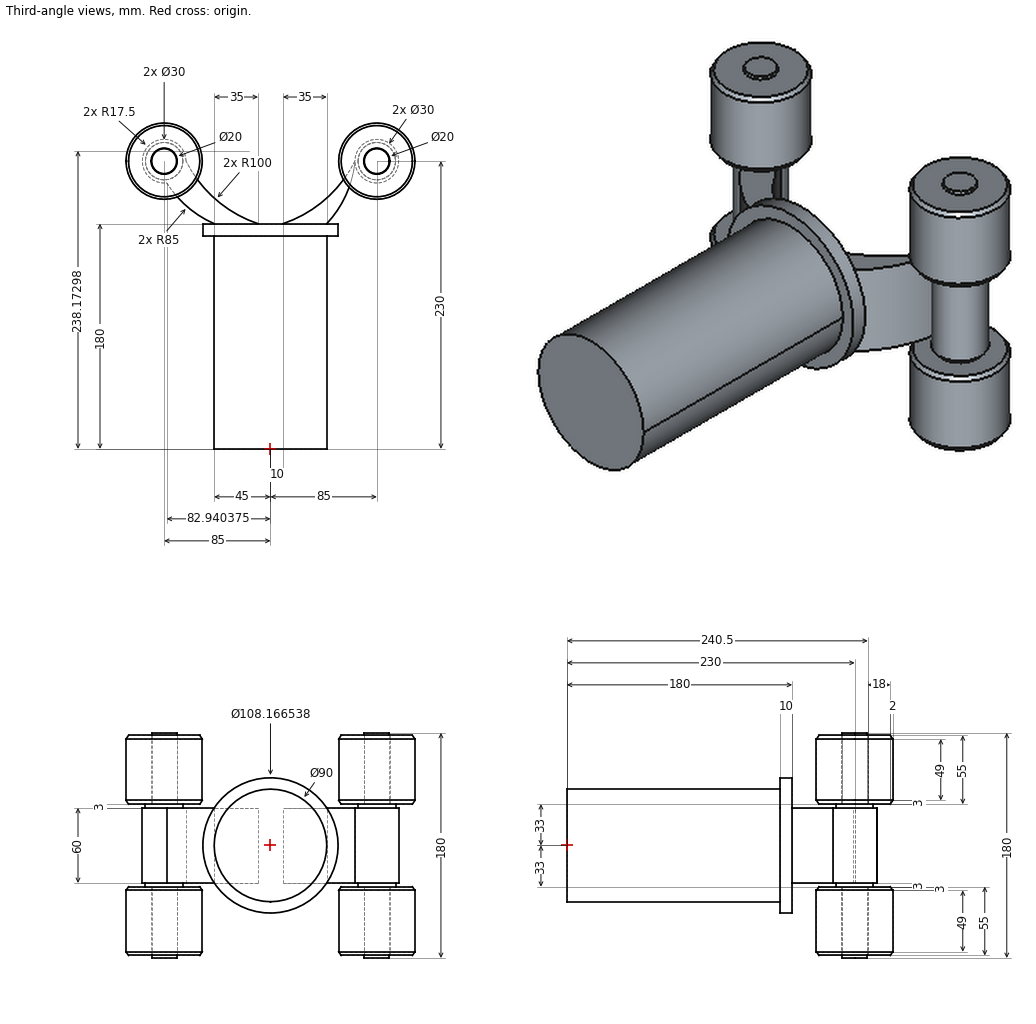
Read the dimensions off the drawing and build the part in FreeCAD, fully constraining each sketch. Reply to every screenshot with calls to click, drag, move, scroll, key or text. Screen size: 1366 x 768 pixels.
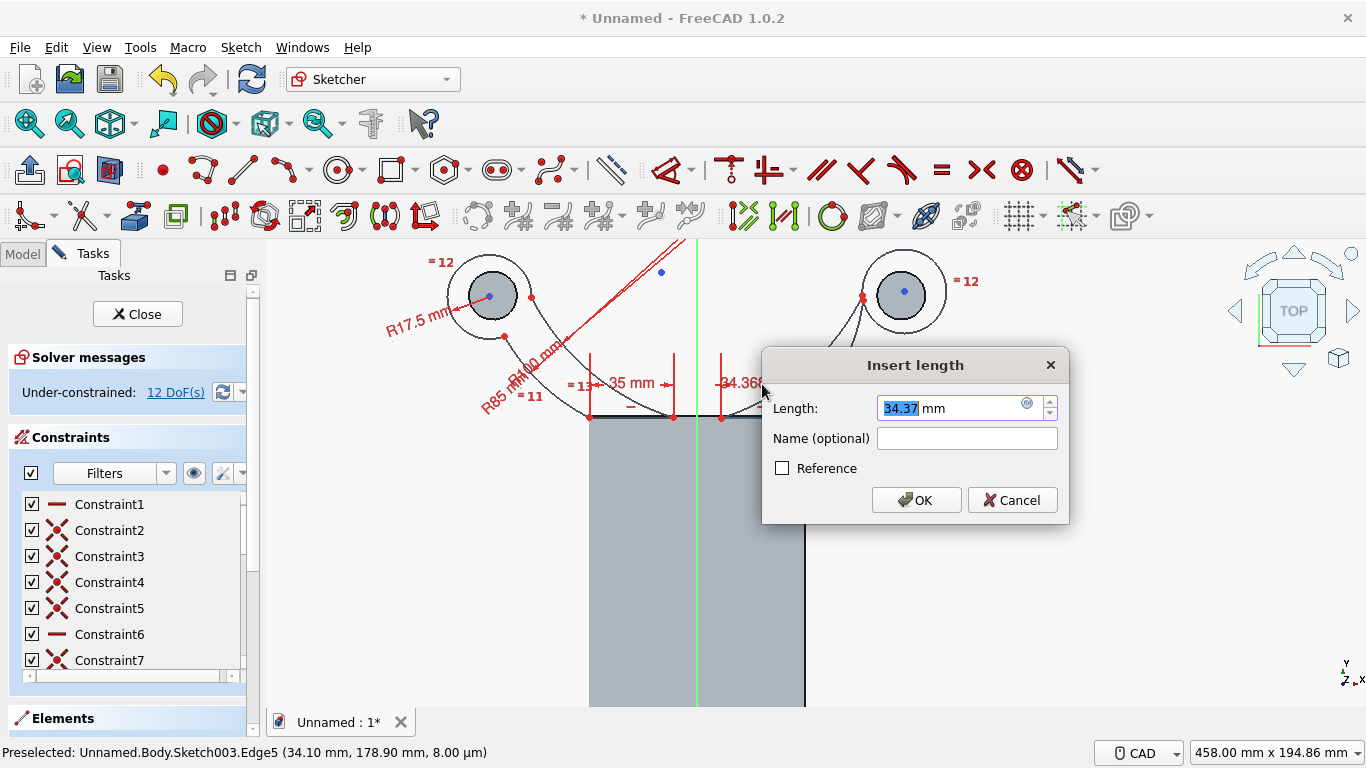
text(35)
key(Return)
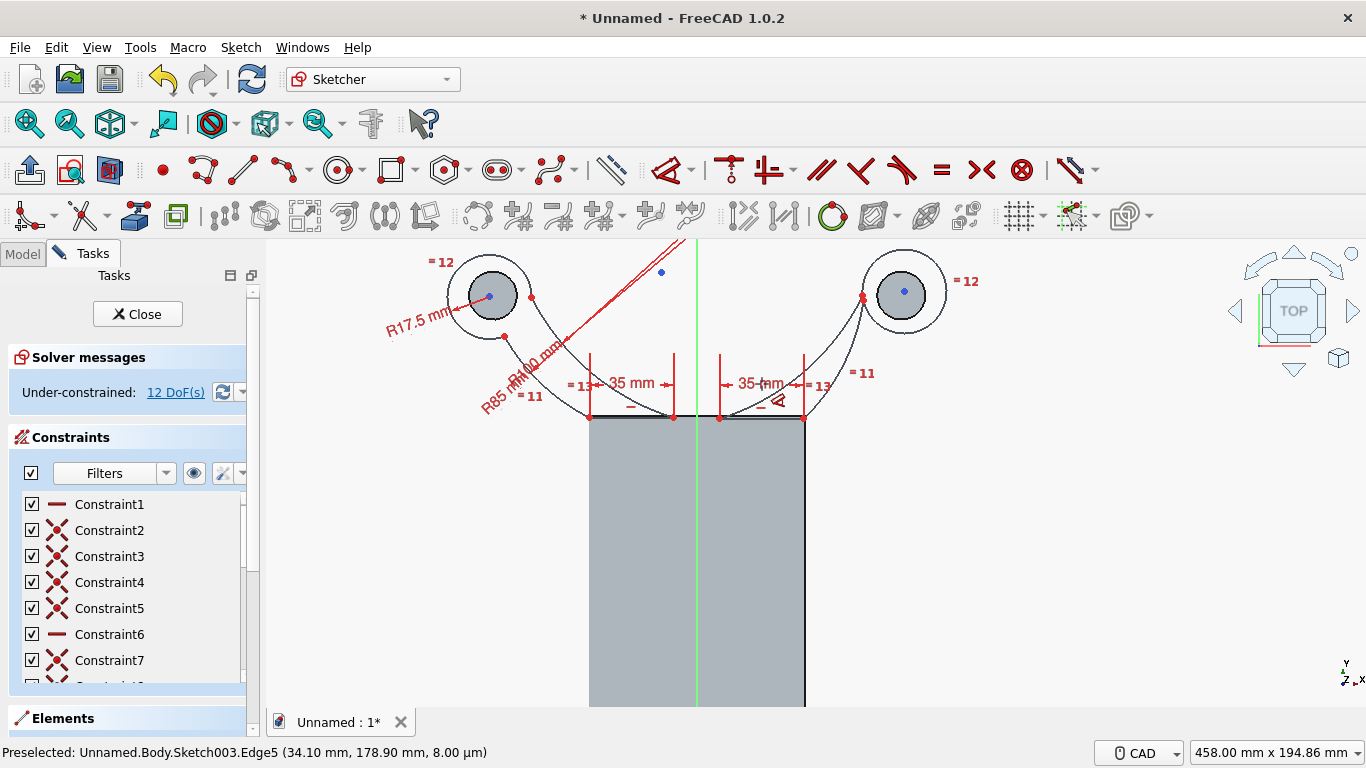
click(590, 418)
click(643, 360)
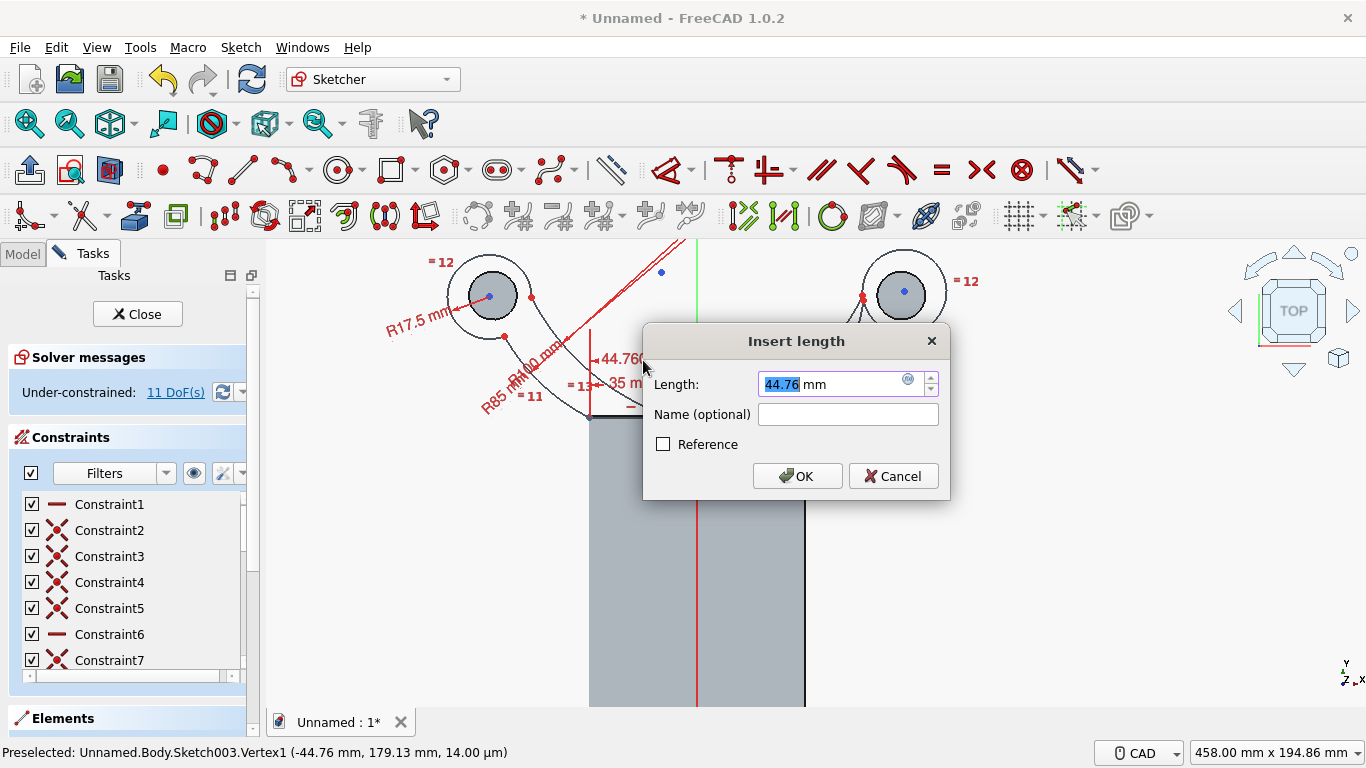
text(45)
key(Return)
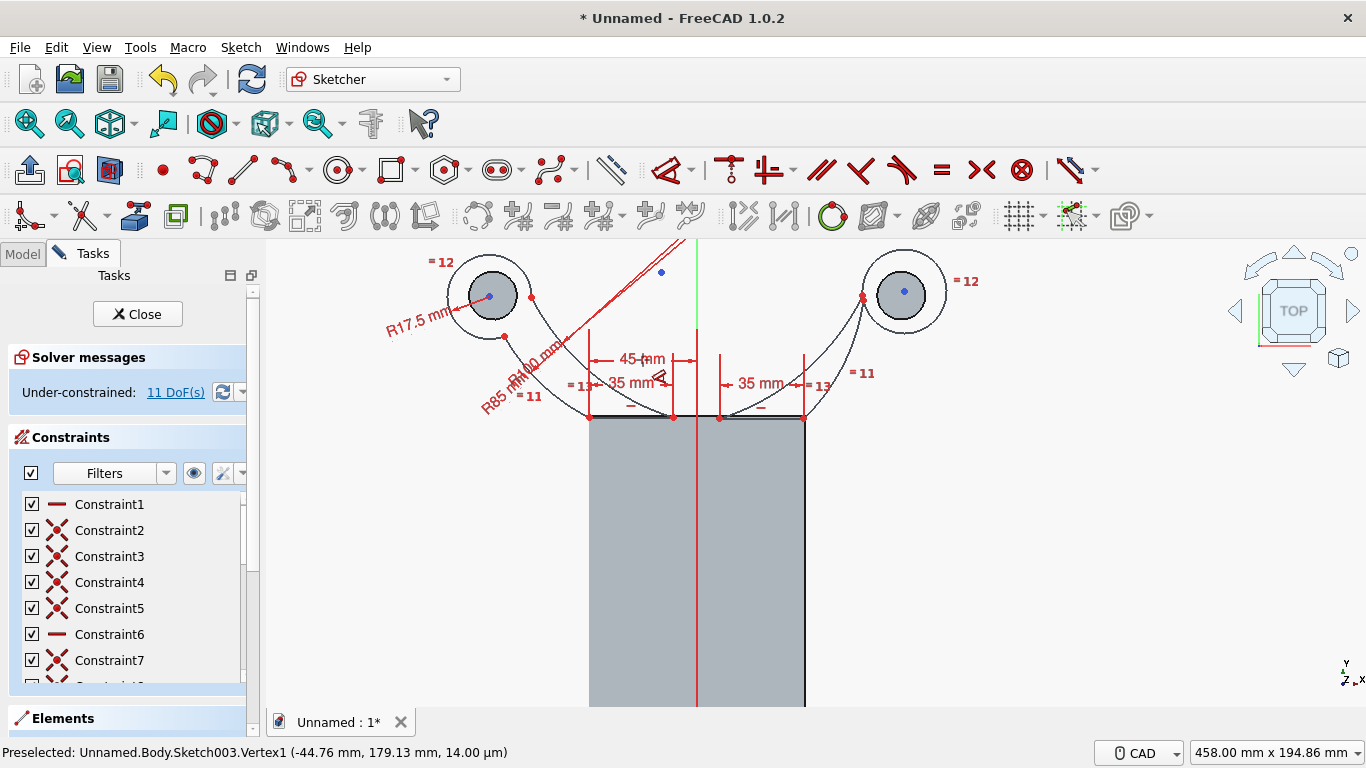
scroll(720, 419, up, 3)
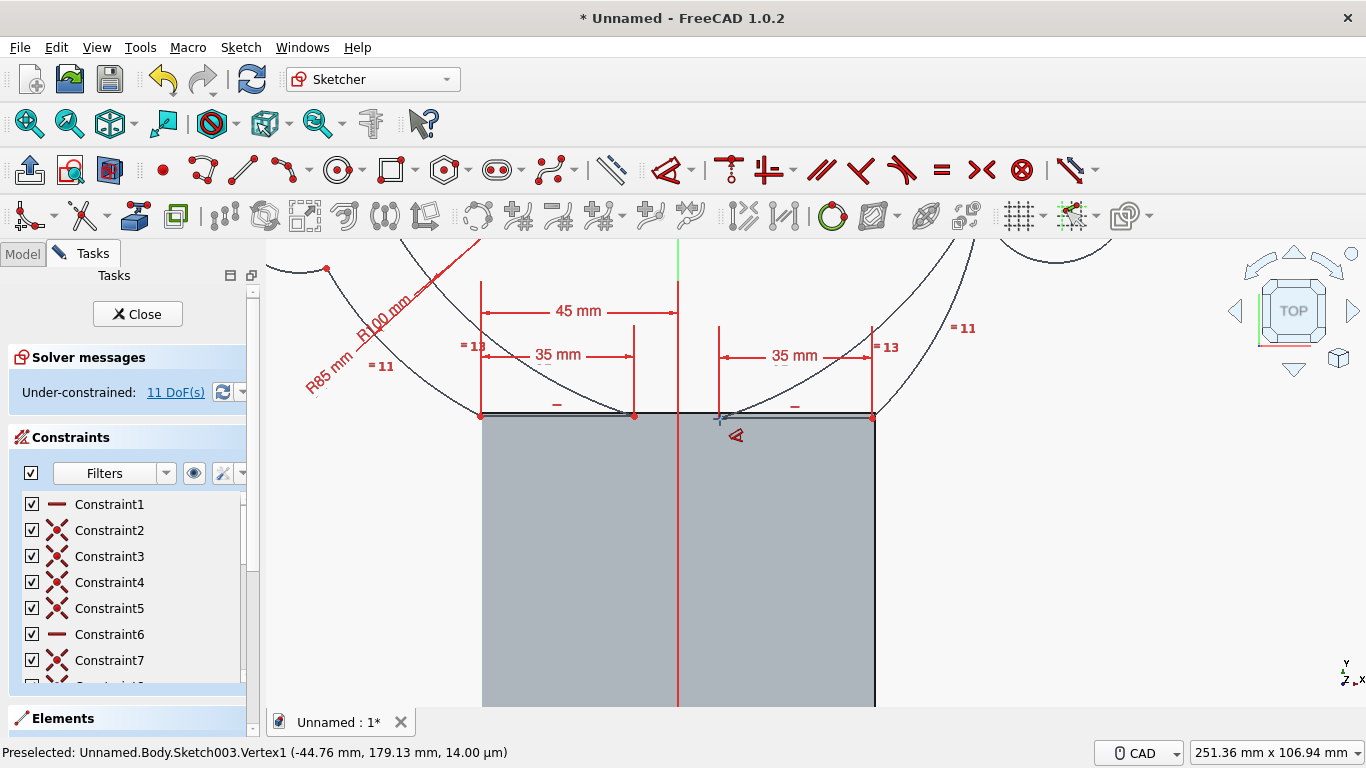
click(719, 418)
click(699, 384)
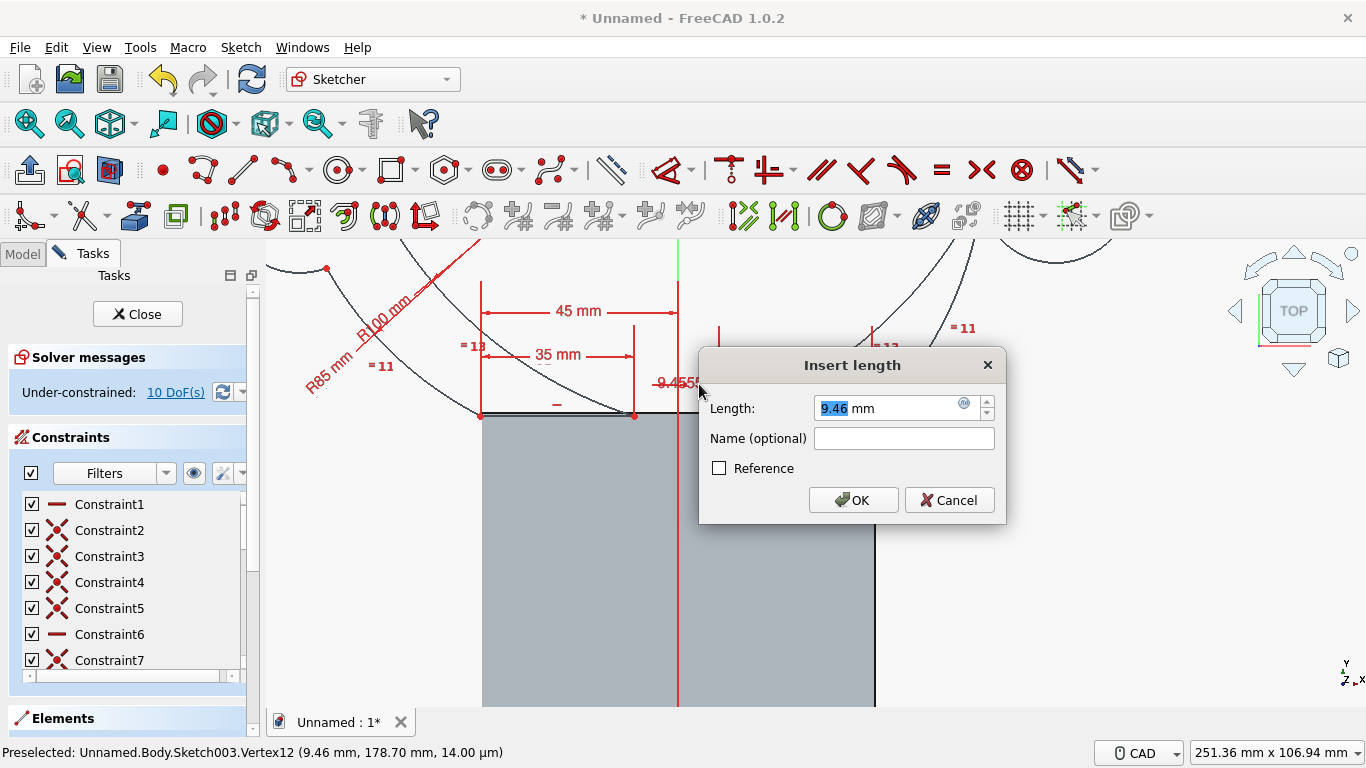
text(10)
key(Return)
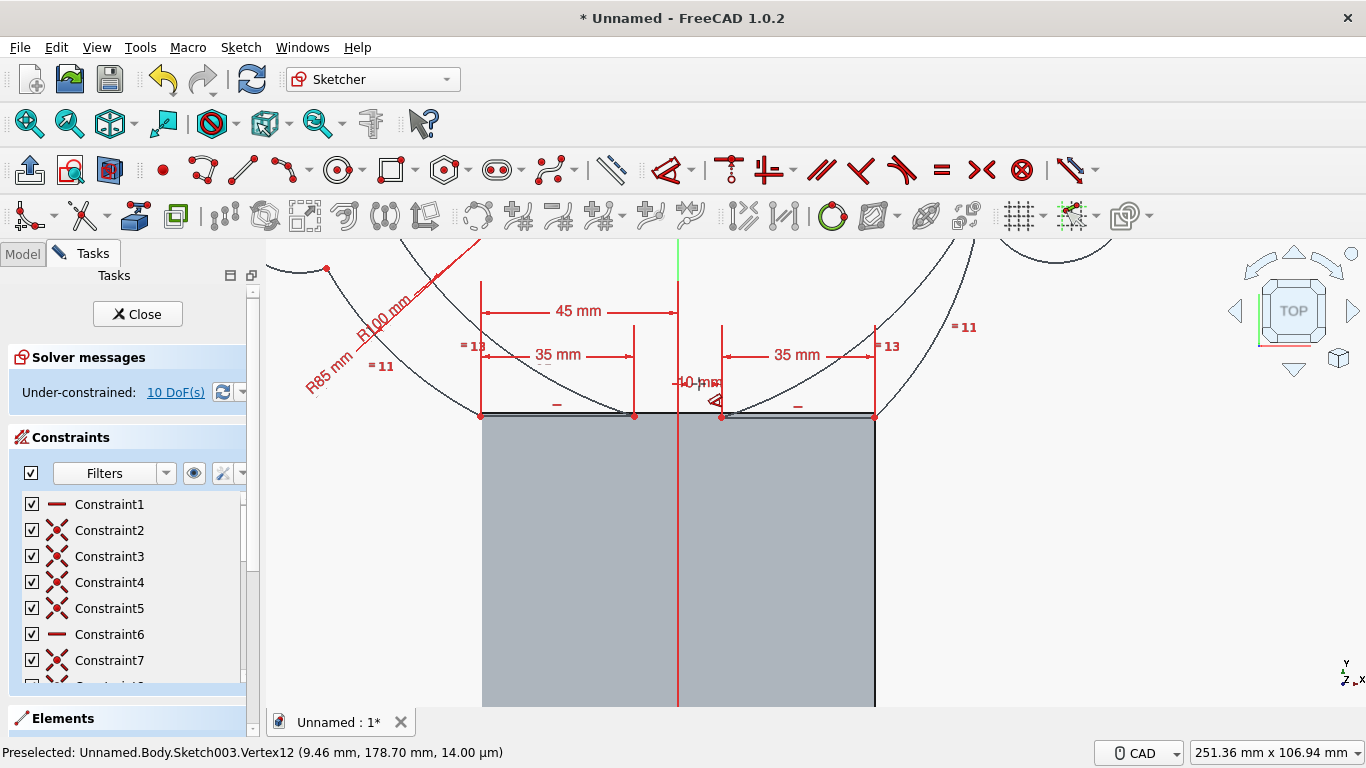
scroll(773, 387, down, 6)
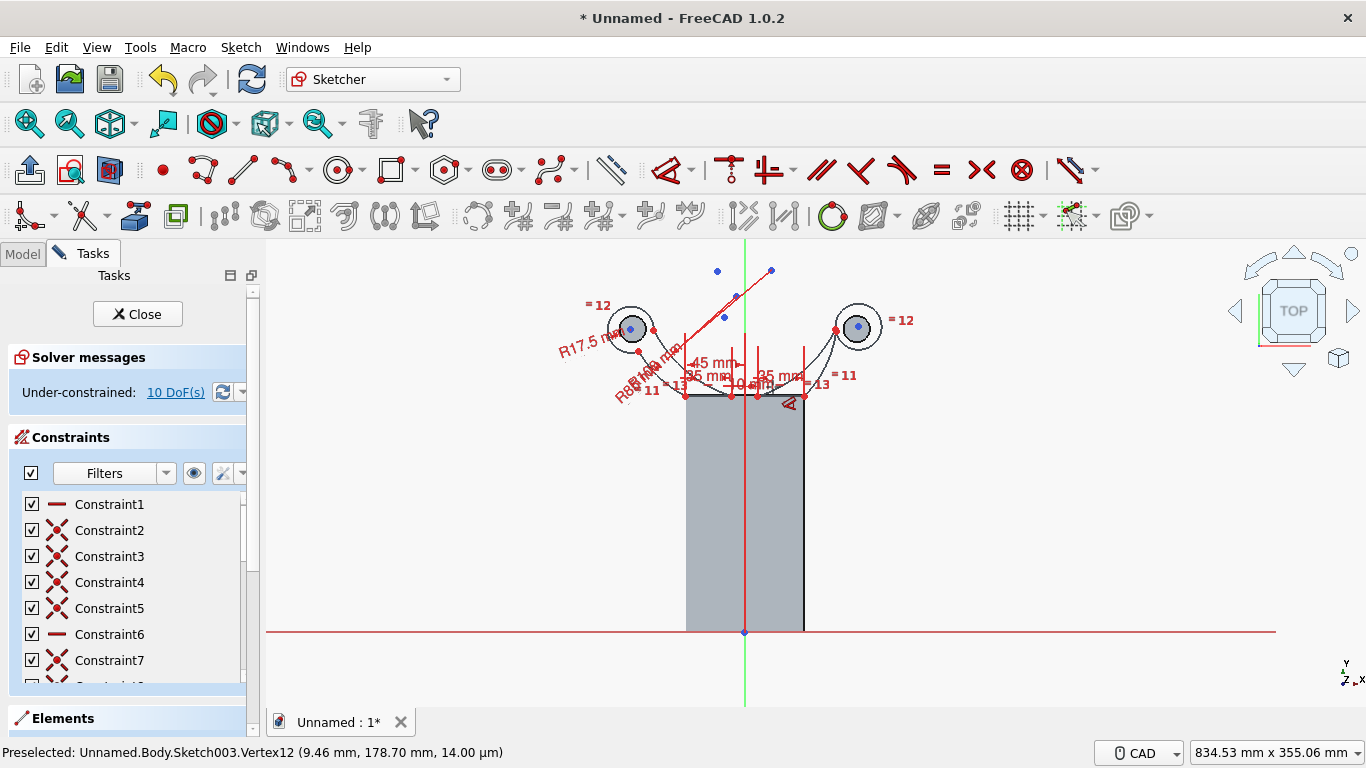
click(631, 330)
click(688, 666)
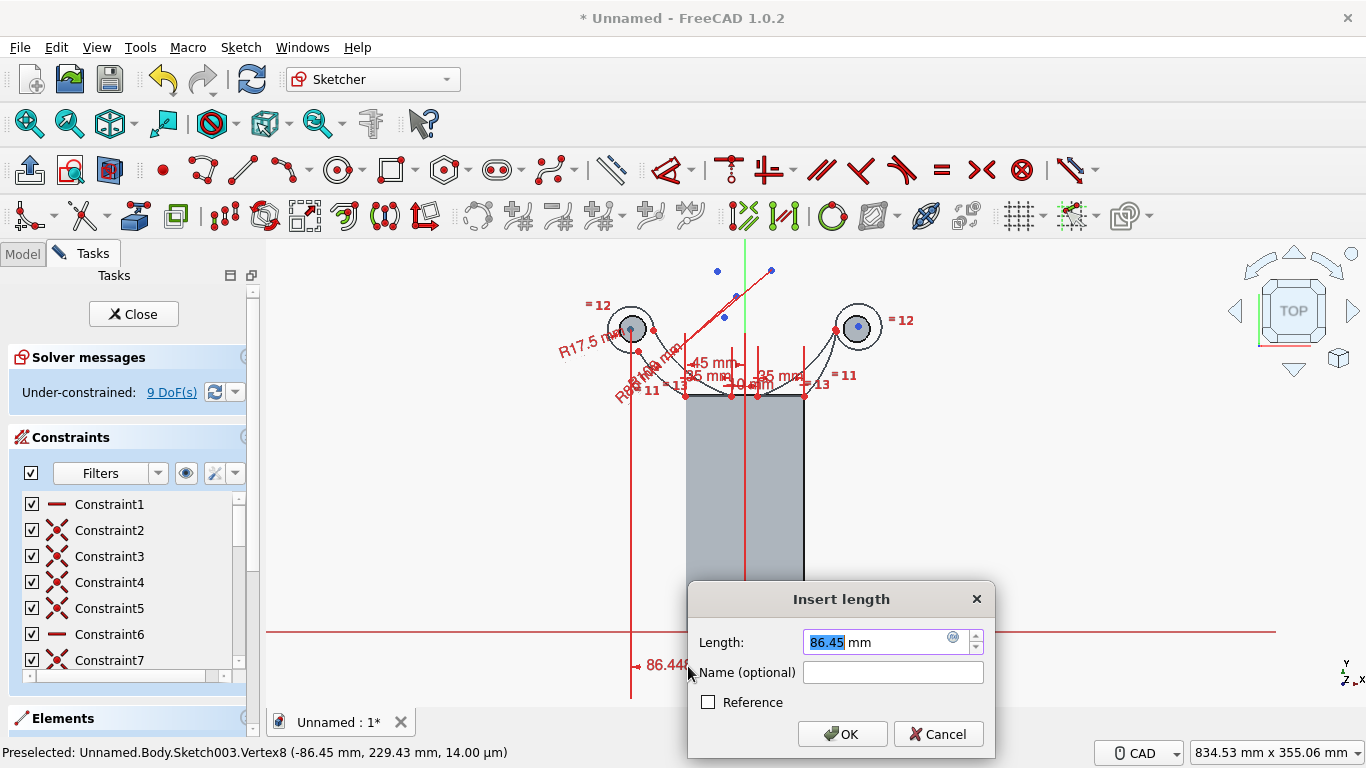
text(85)
key(Return)